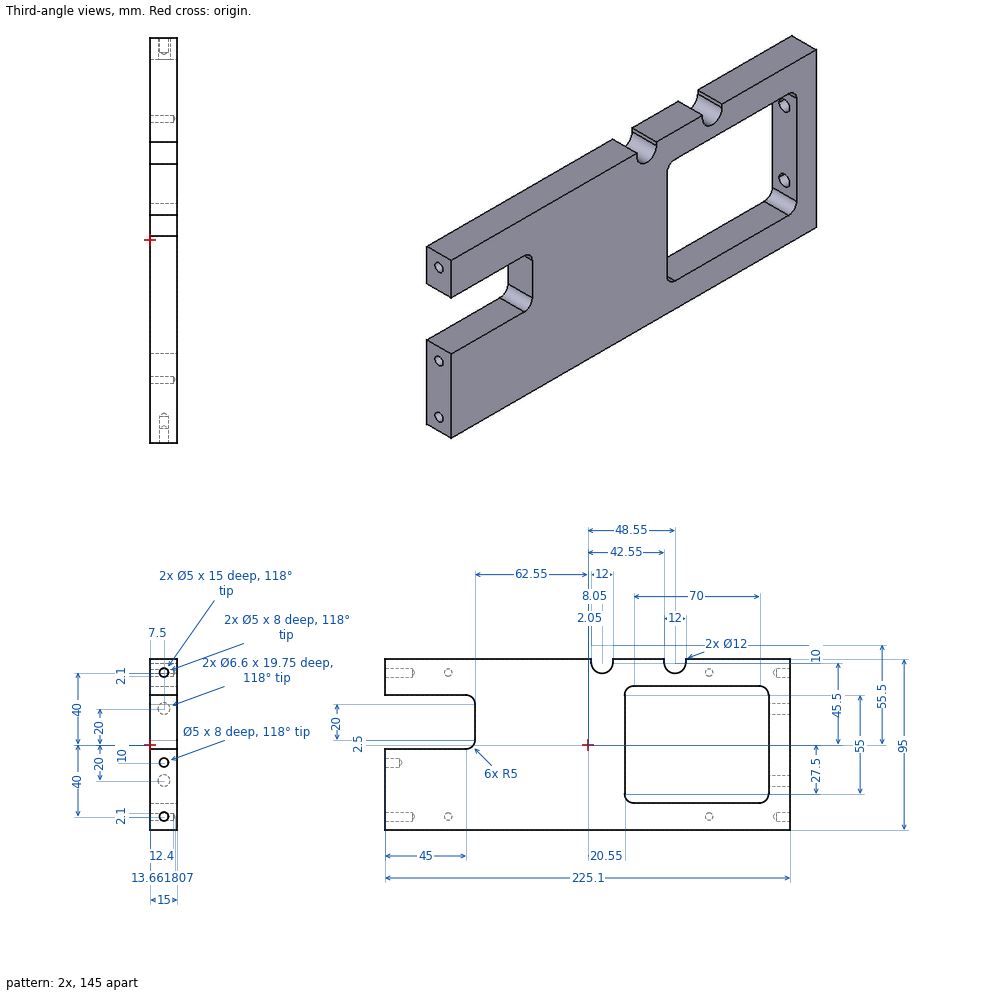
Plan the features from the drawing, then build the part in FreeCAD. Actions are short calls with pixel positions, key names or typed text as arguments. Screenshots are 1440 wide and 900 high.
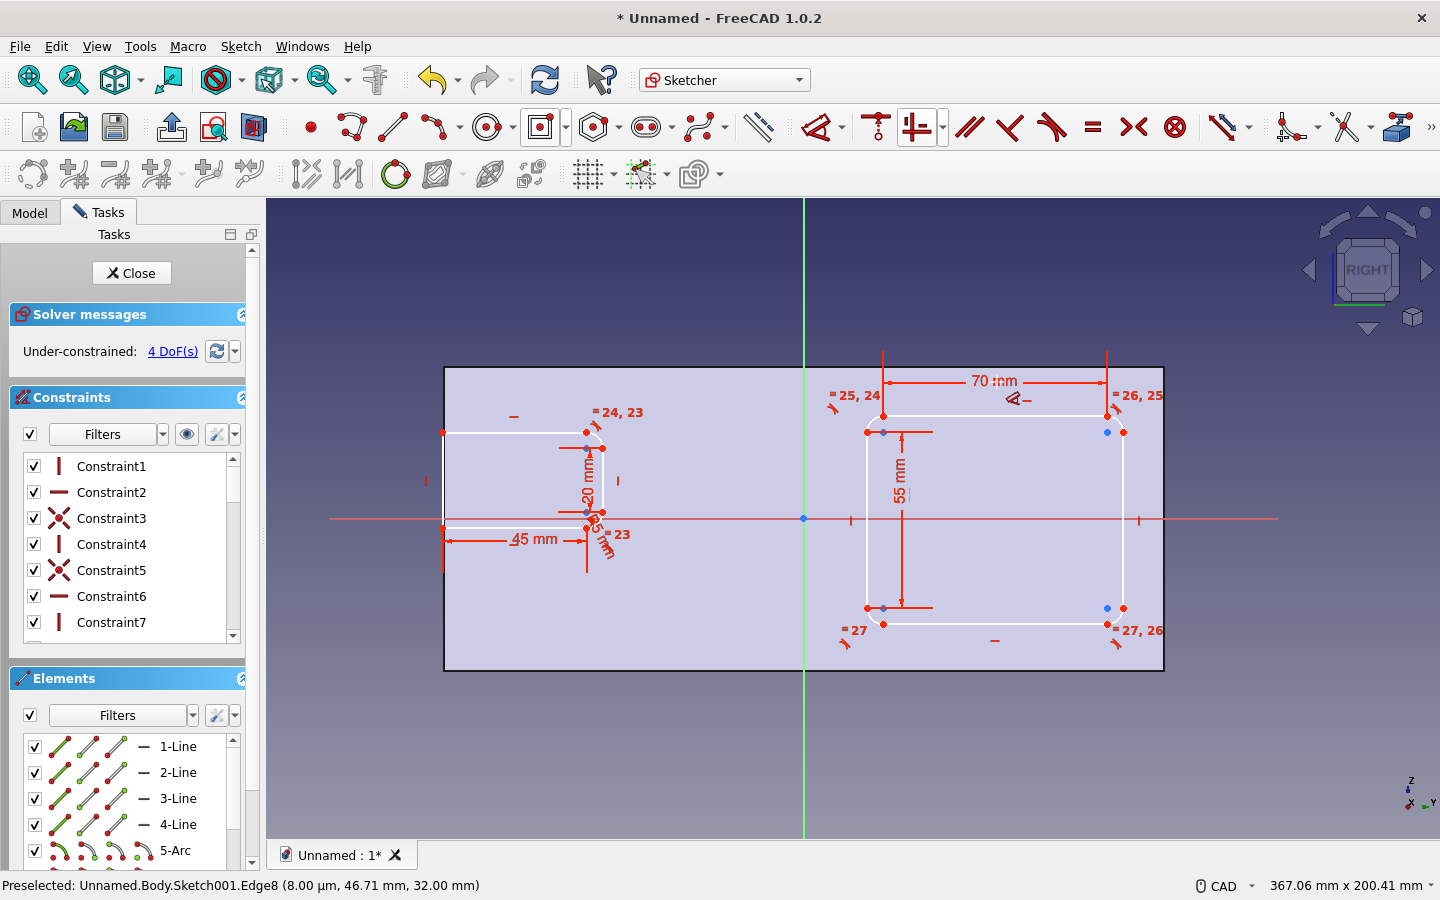
scroll(603, 512, up, 9)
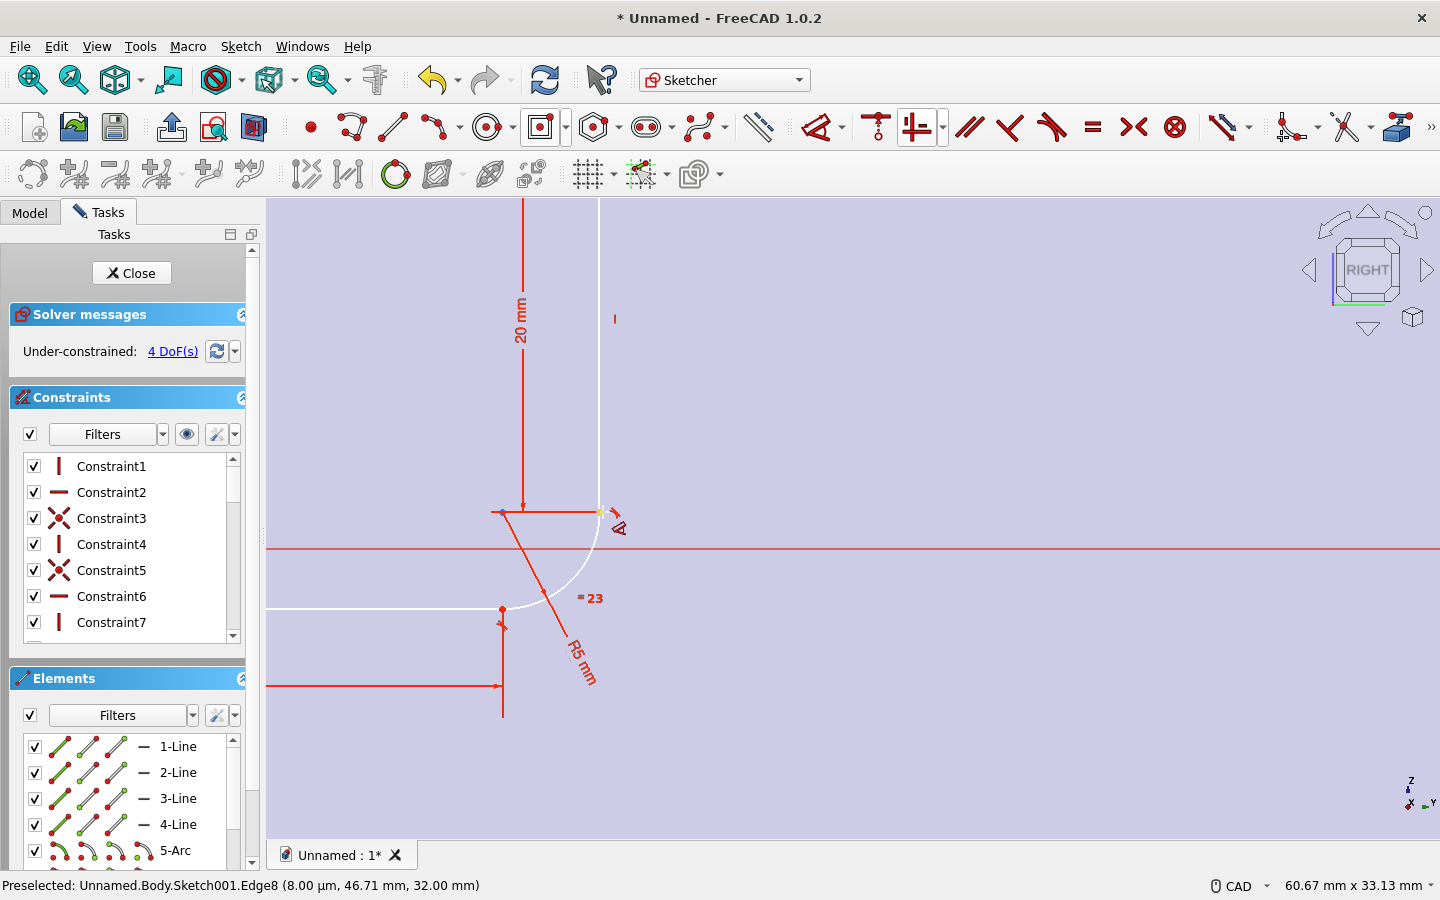
click(599, 512)
click(565, 531)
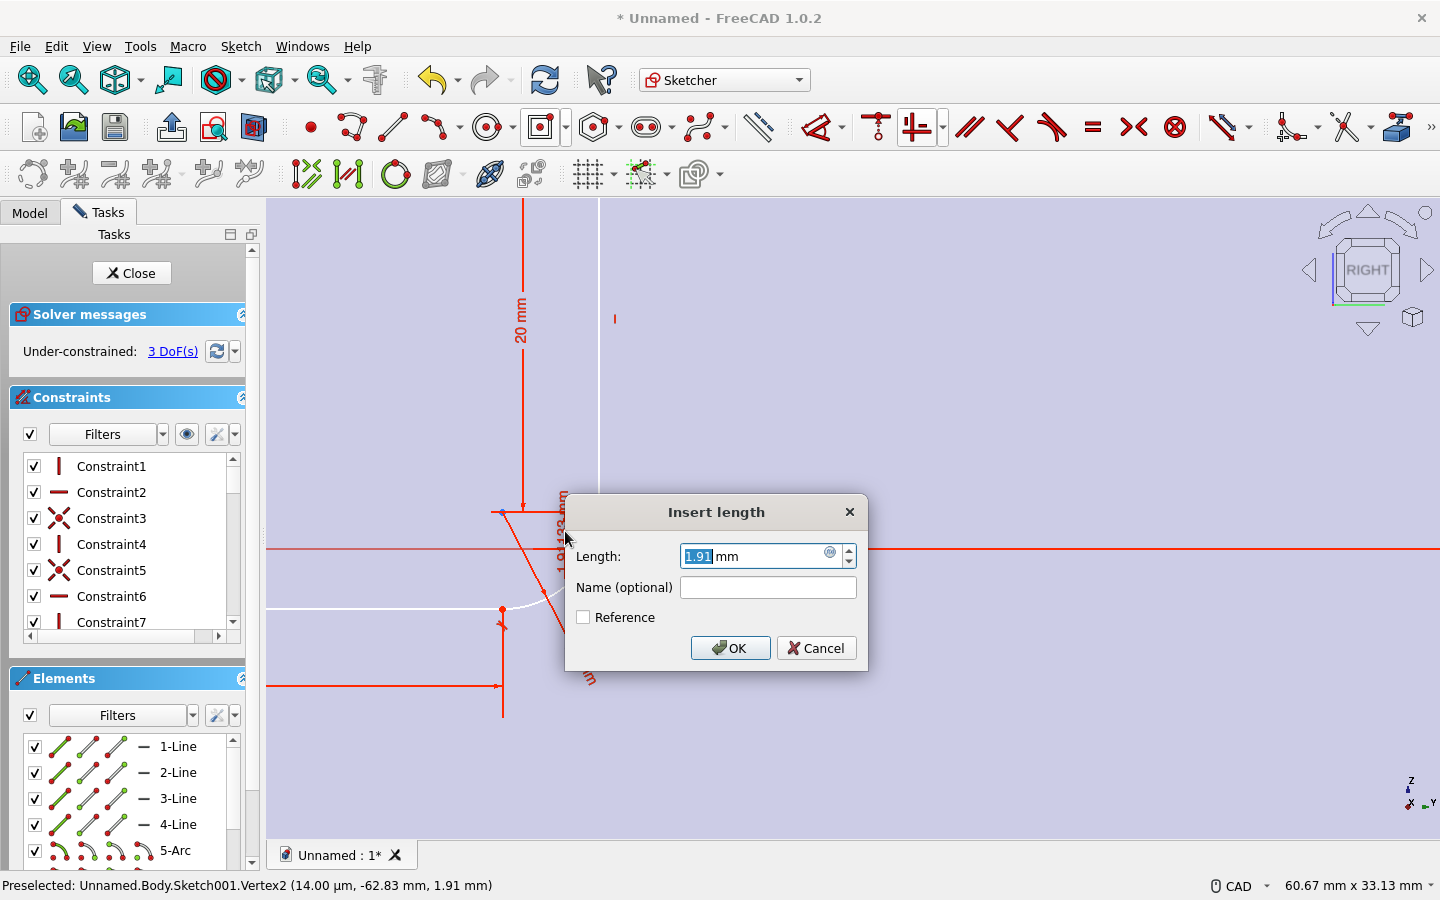
text(2.5)
key(Return)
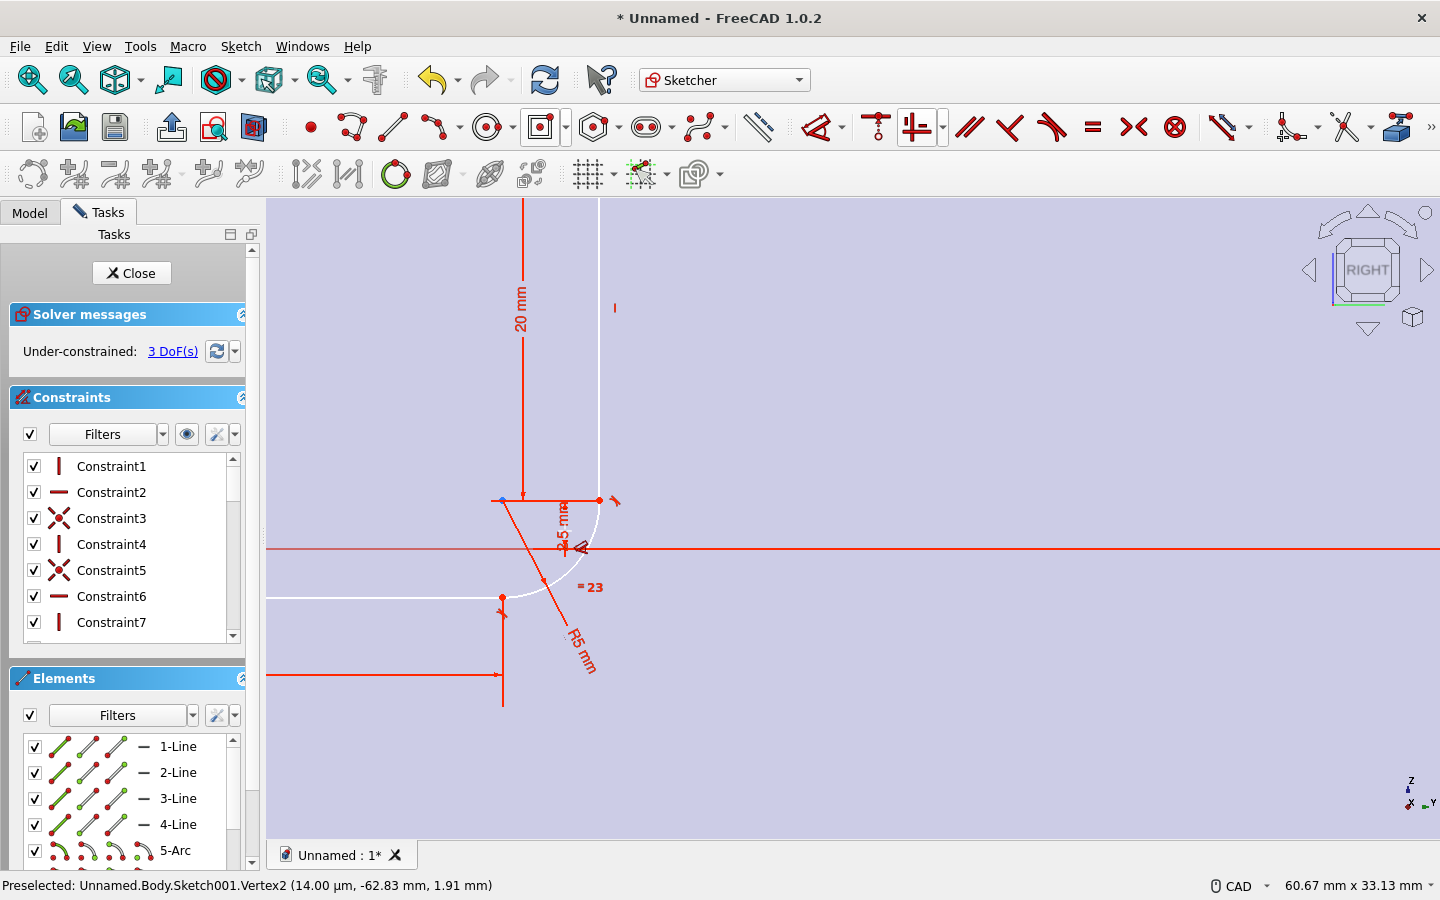
scroll(603, 512, down, 9)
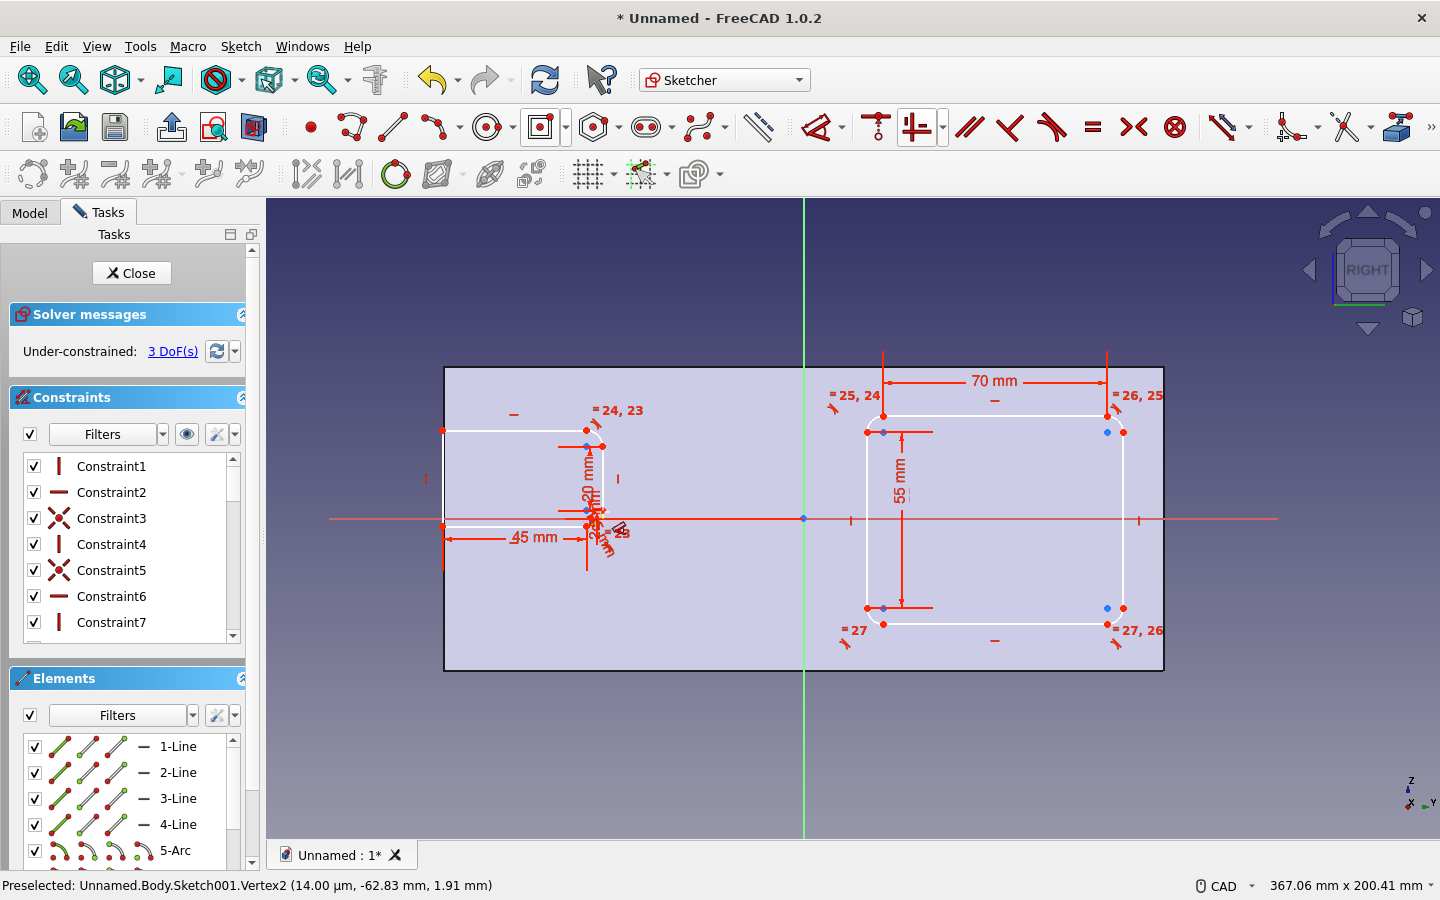
click(867, 608)
click(901, 563)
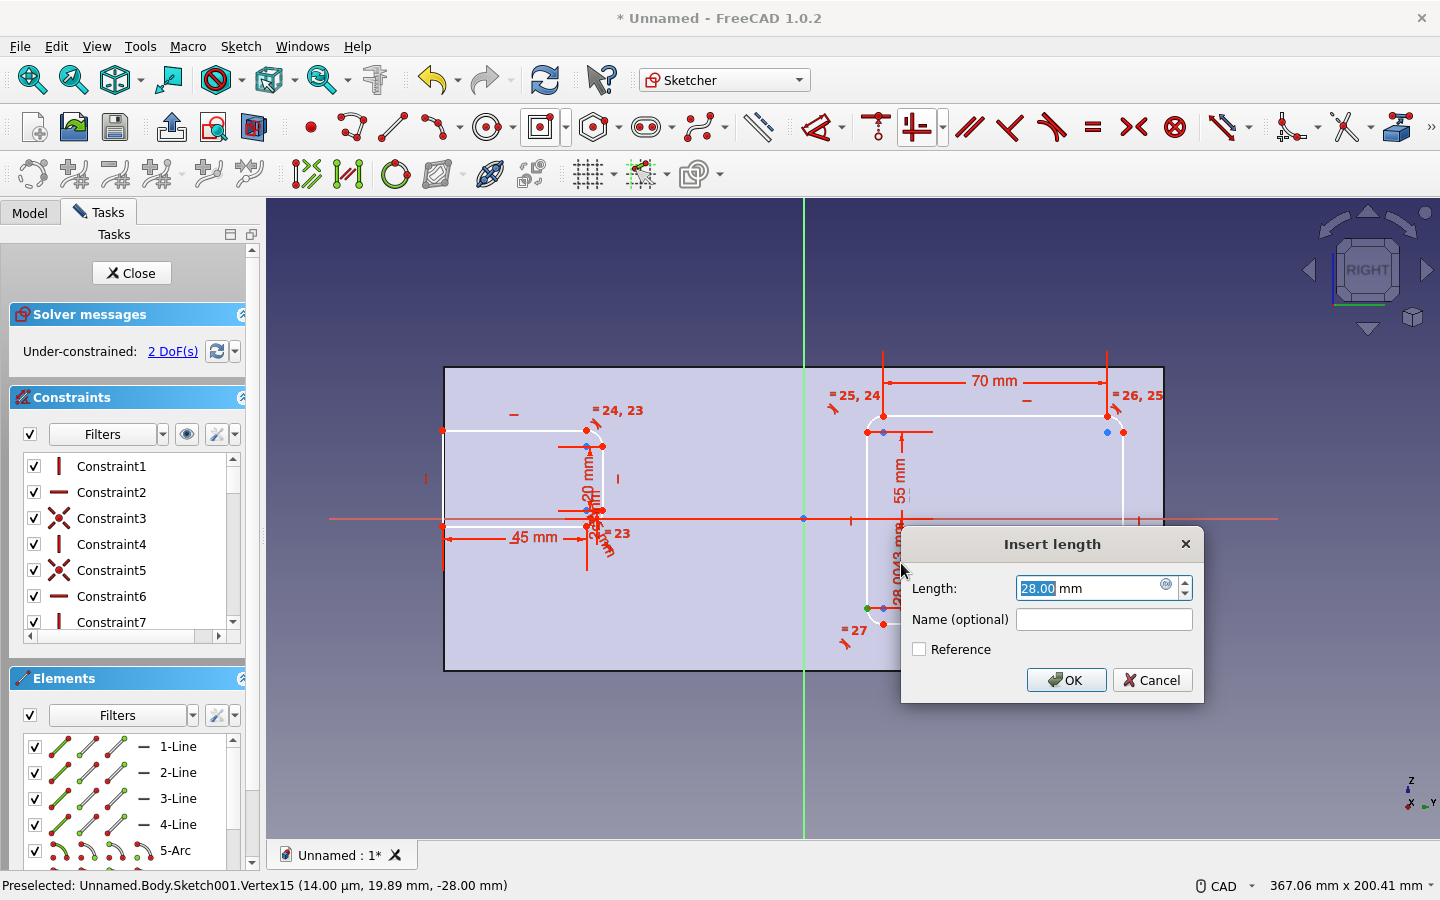
text(27.5)
key(Return)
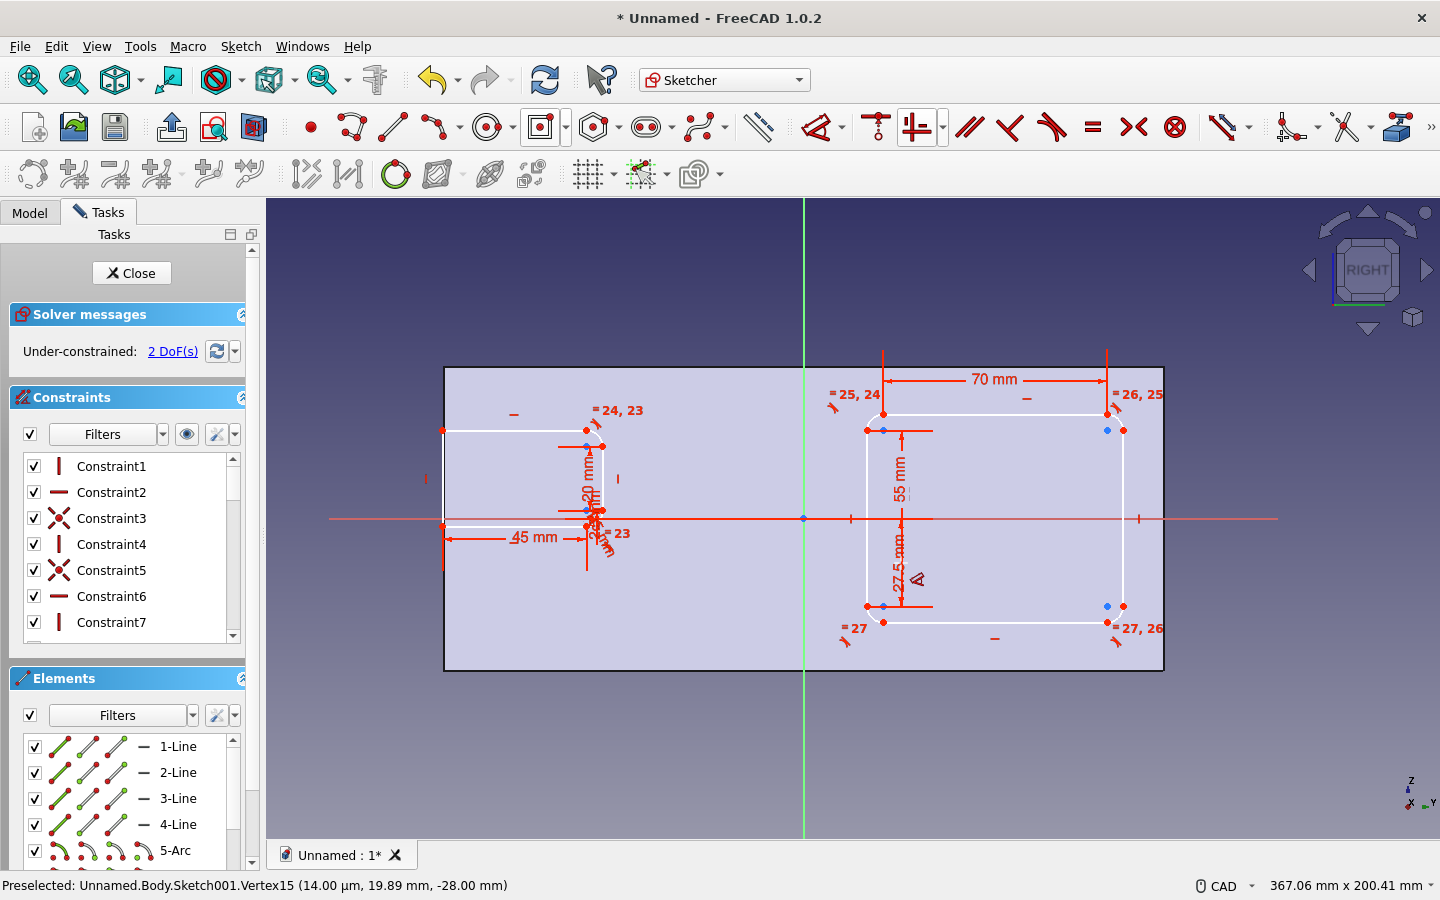
click(603, 447)
click(703, 413)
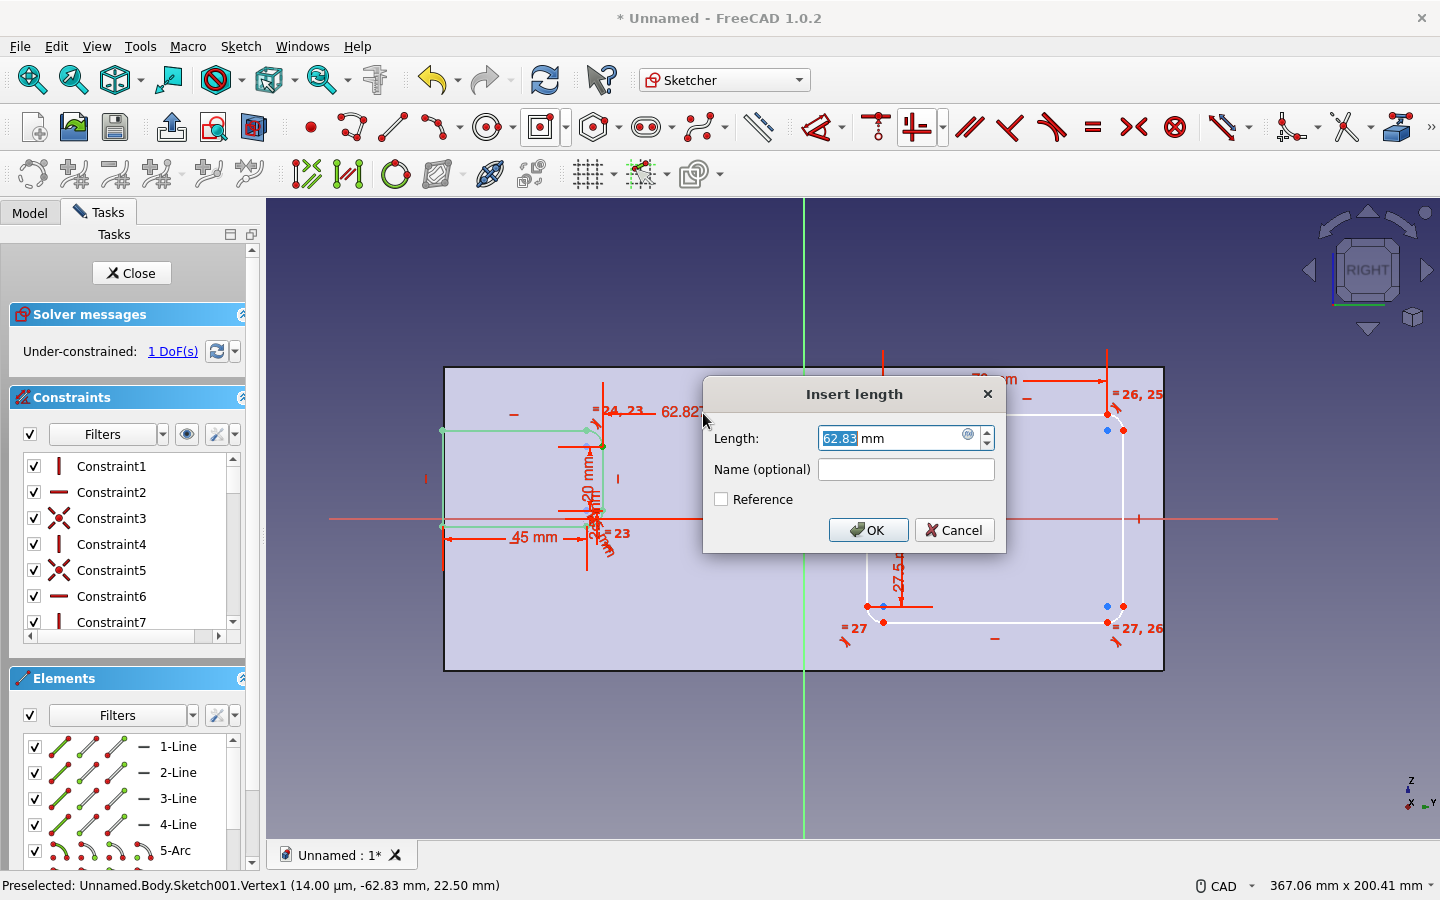
text(62.55)
key(Return)